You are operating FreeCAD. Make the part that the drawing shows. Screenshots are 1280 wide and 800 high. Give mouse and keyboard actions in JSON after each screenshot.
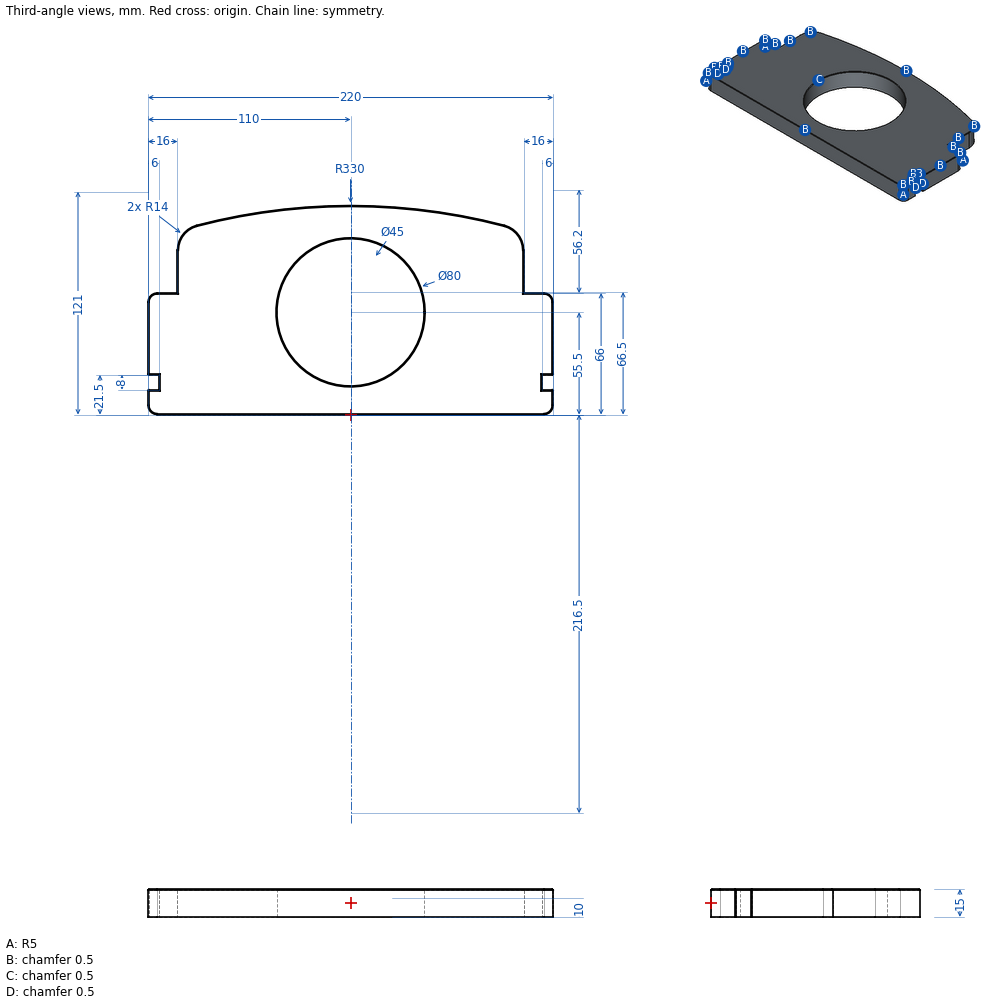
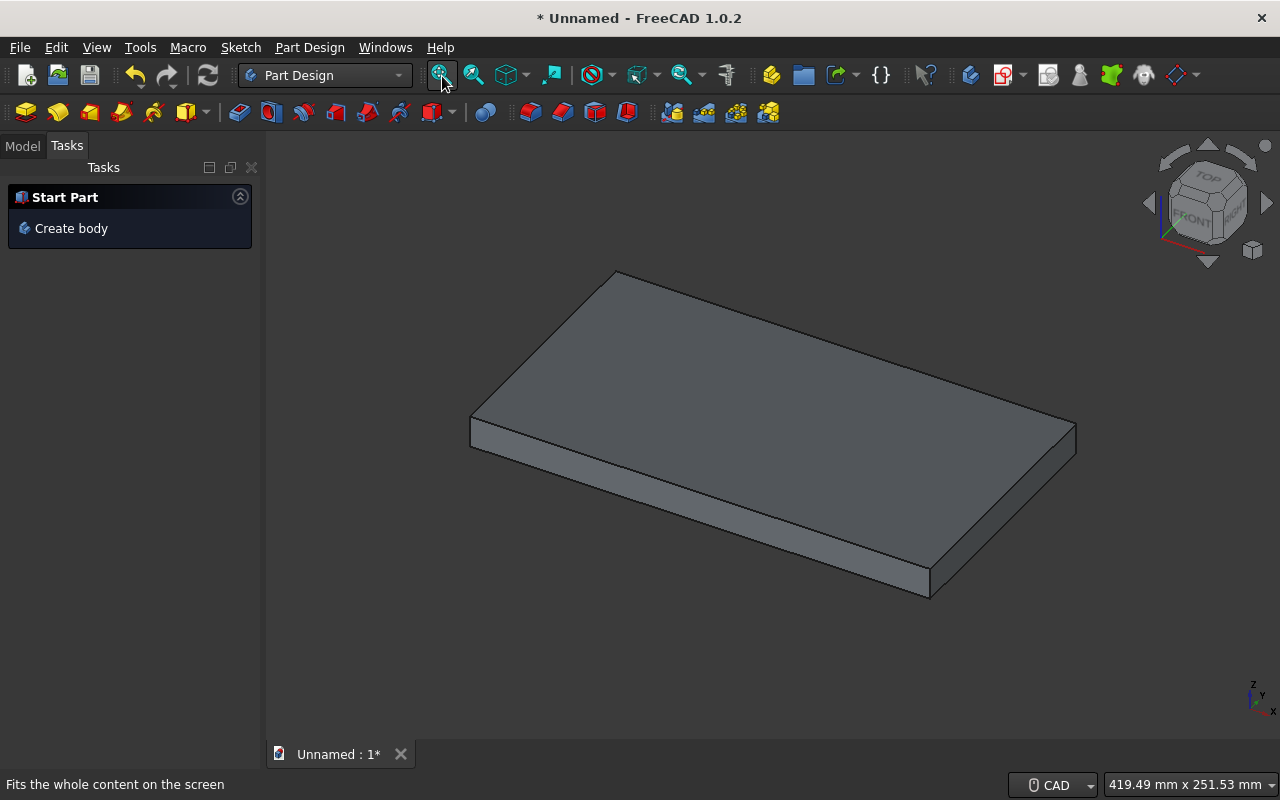
{"action": "left_click", "coordinate": [839, 441]}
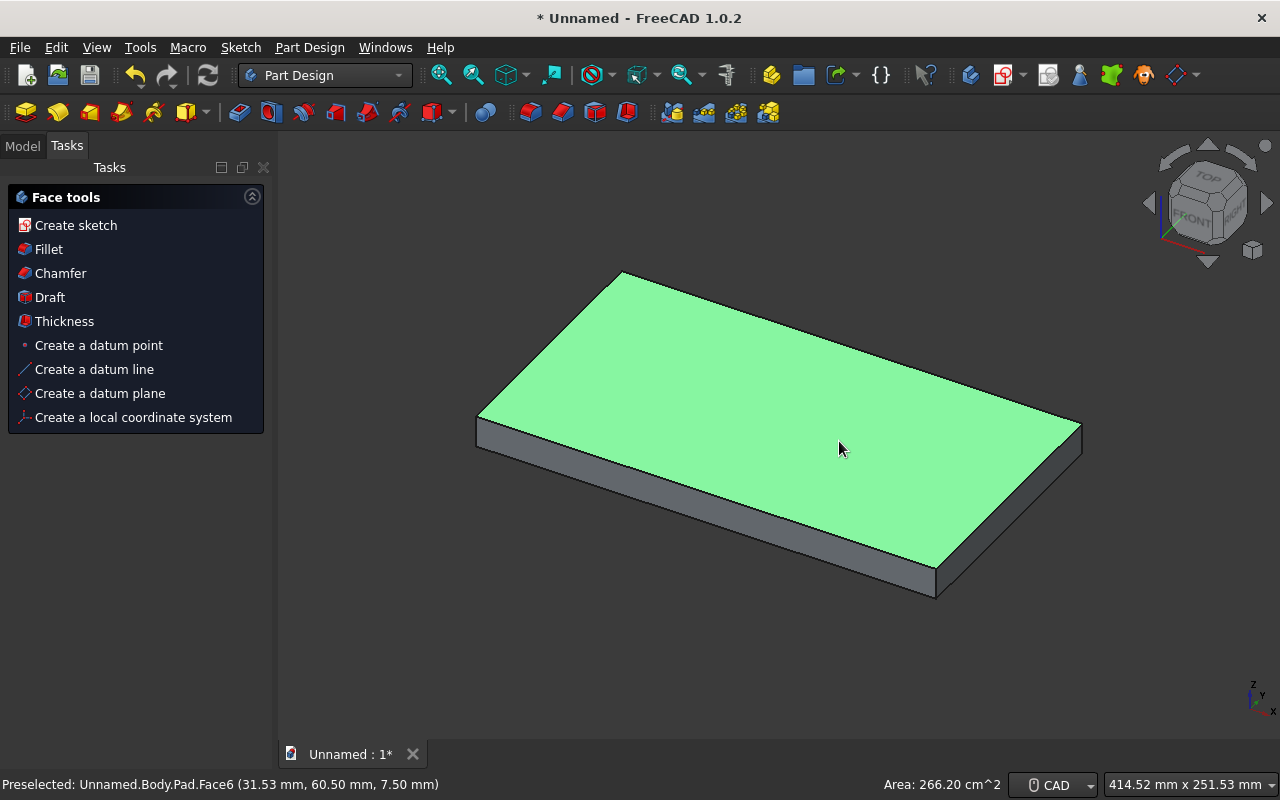
{"action": "left_click", "coordinate": [1004, 76]}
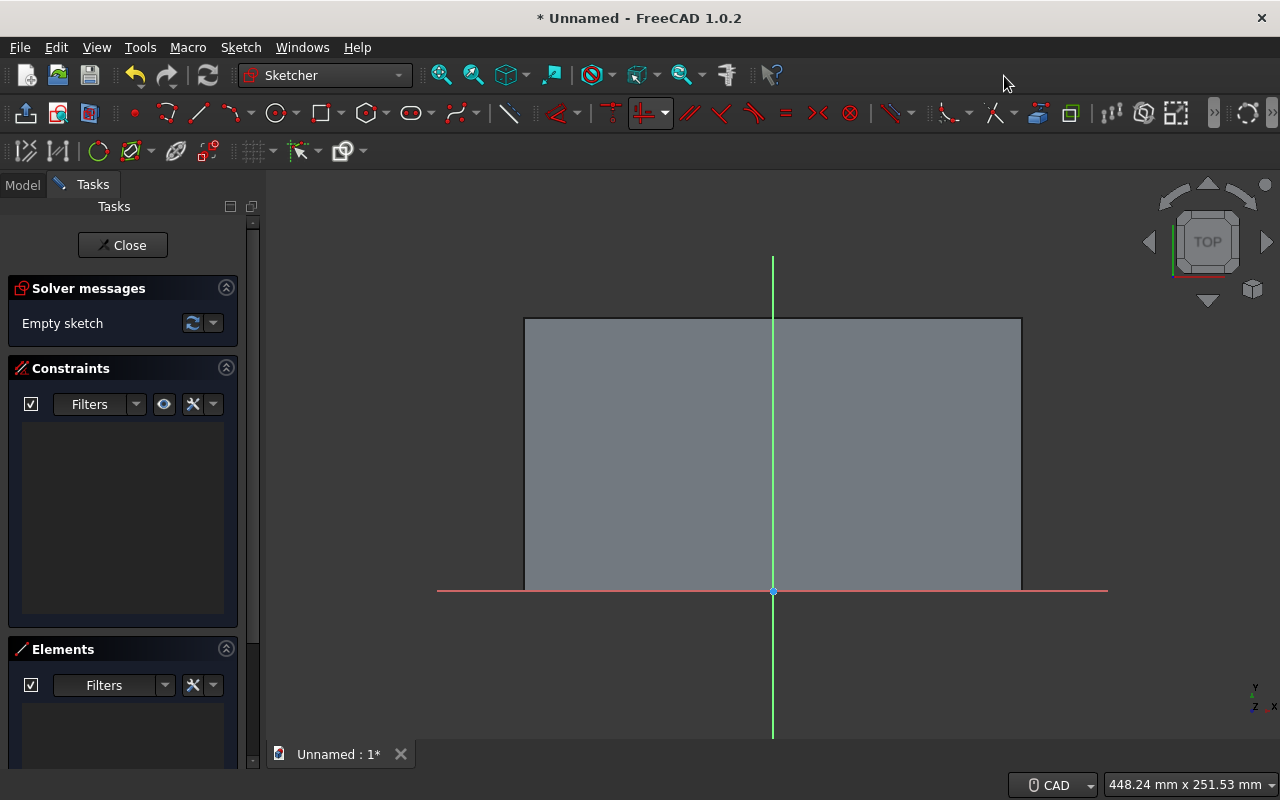
{"action": "left_click", "coordinate": [322, 114]}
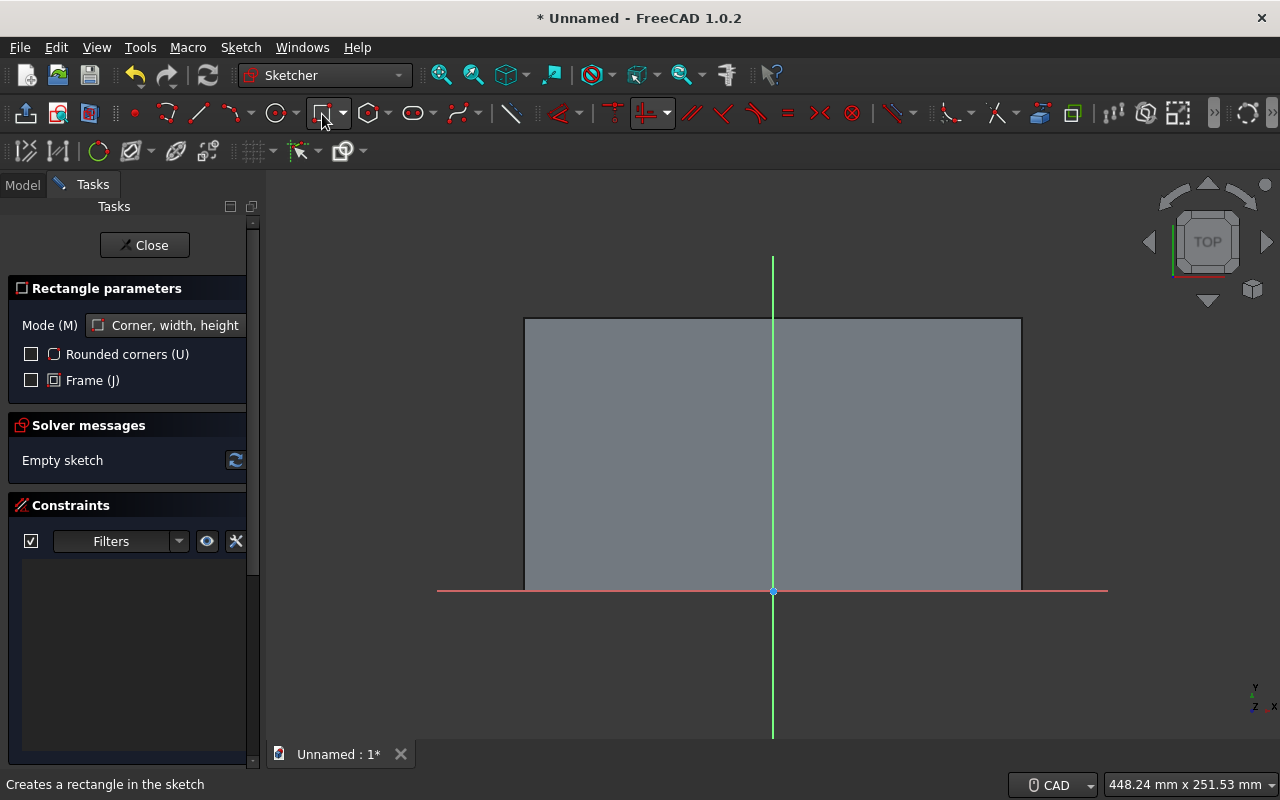
{"action": "left_click", "coordinate": [524, 543]}
{"action": "mouse_move", "coordinate": [538, 561]}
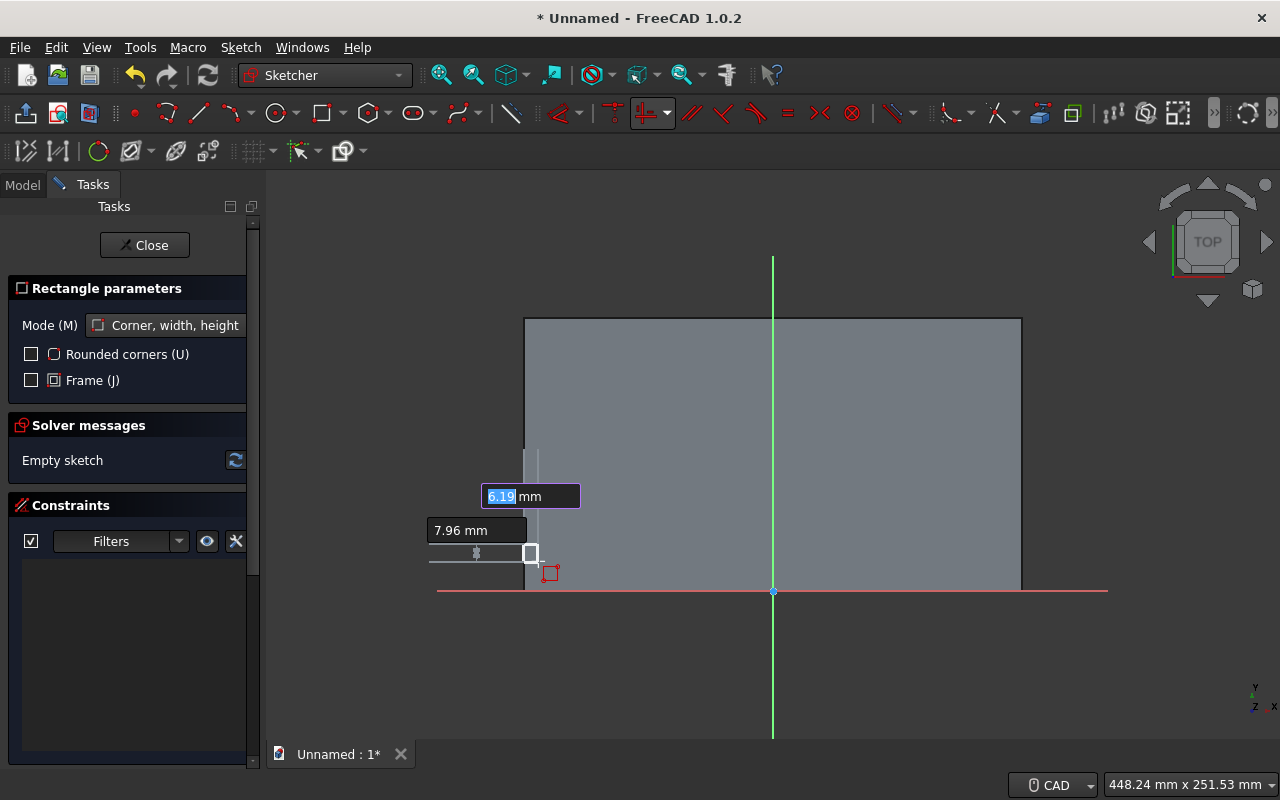
{"action": "type", "text": "6"}
{"action": "key", "text": "Tab"}
{"action": "type", "text": "8"}
{"action": "key", "text": "Return"}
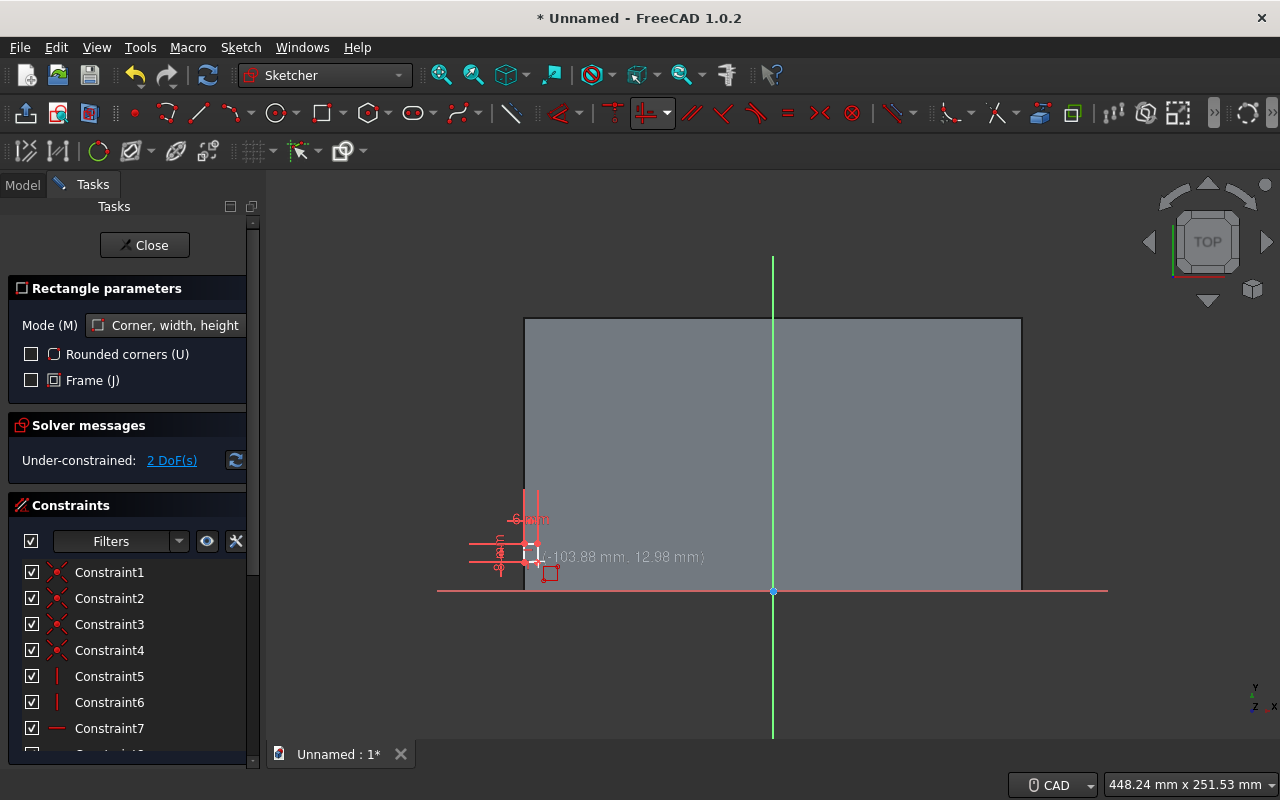
{"action": "left_click", "coordinate": [1008, 543]}
{"action": "mouse_move", "coordinate": [1022, 561]}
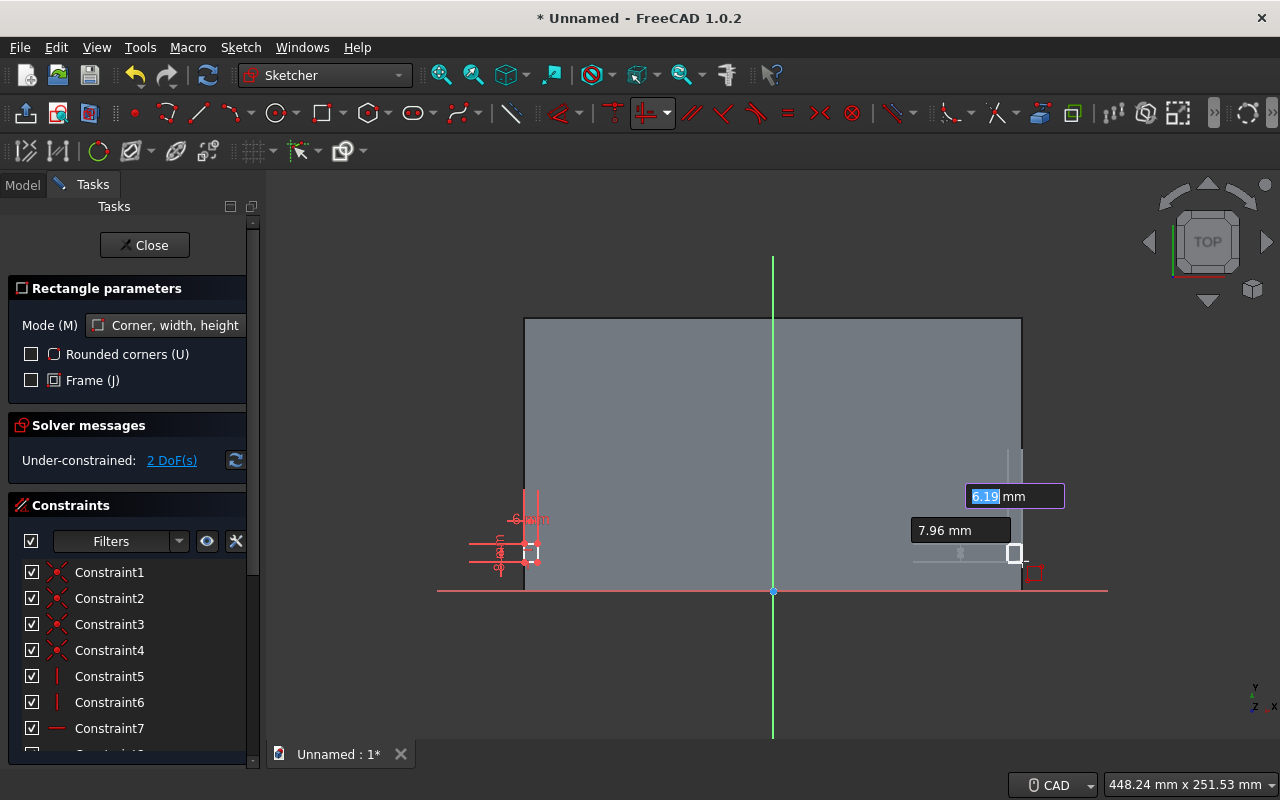
{"action": "type", "text": "6"}
{"action": "key", "text": "Tab"}
{"action": "type", "text": "8"}
{"action": "key", "text": "Return"}
{"action": "key", "text": "Escape"}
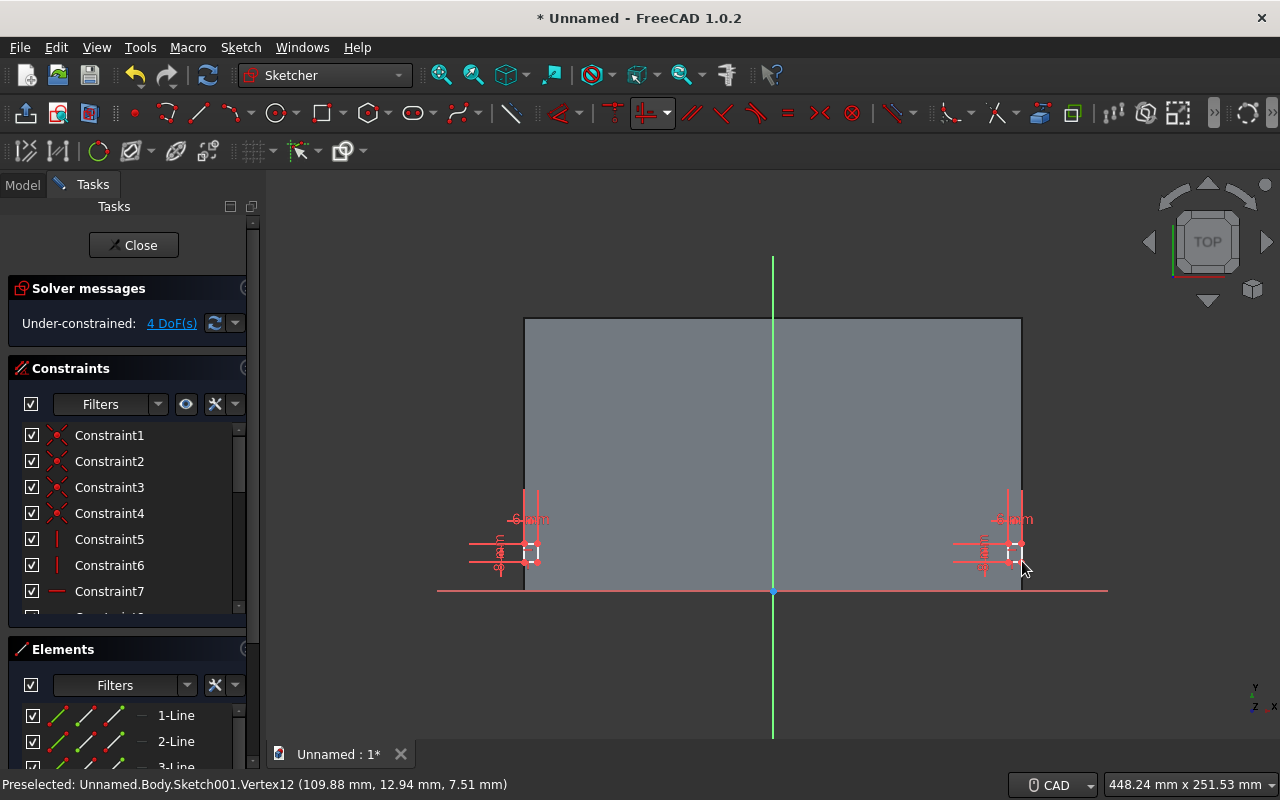
{"action": "left_click", "coordinate": [538, 544]}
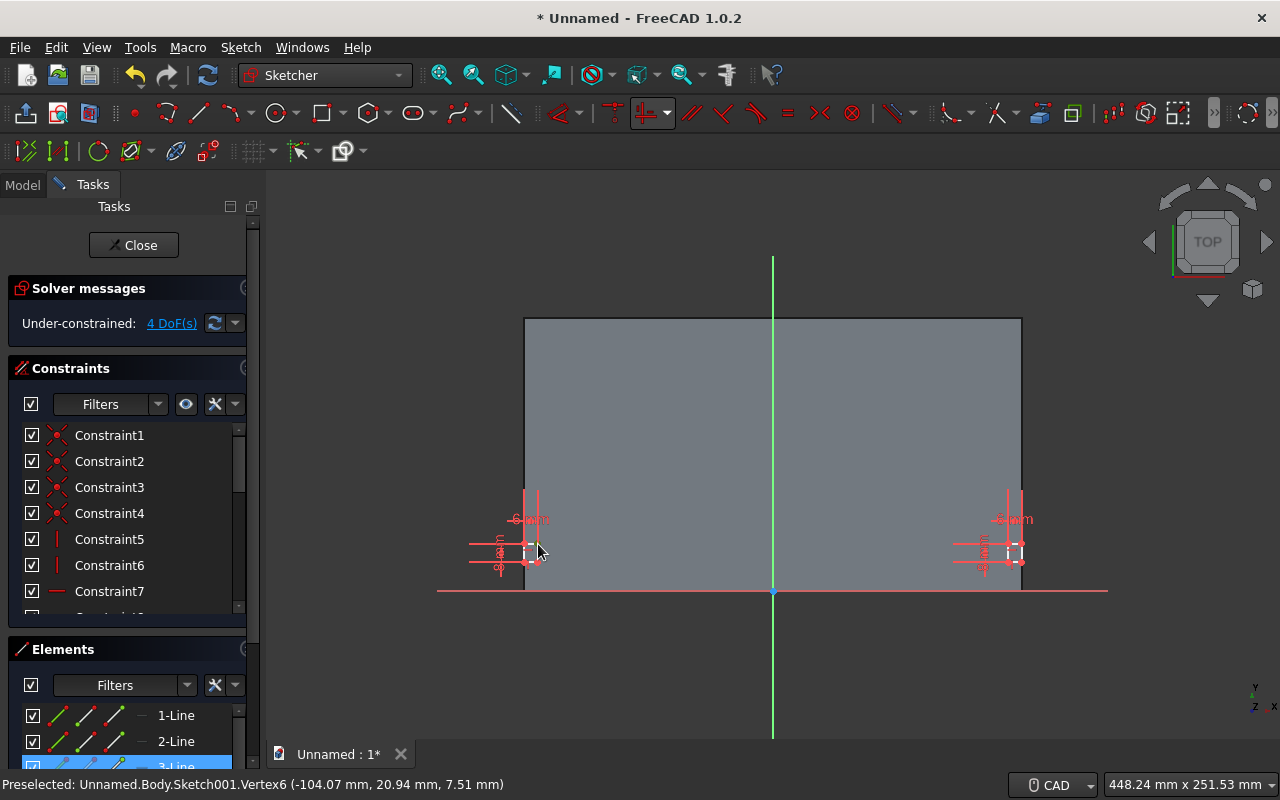
{"action": "left_click", "coordinate": [1008, 544]}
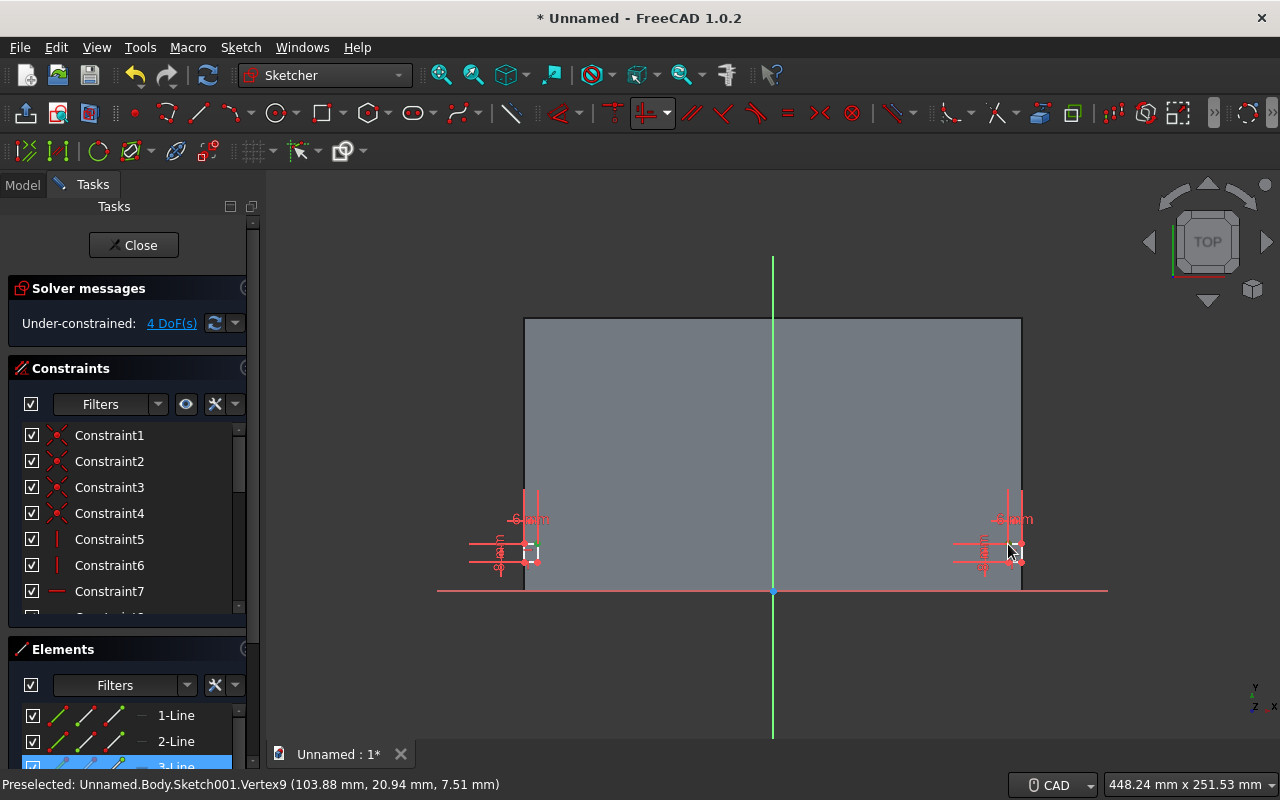
{"action": "left_click", "coordinate": [773, 674]}